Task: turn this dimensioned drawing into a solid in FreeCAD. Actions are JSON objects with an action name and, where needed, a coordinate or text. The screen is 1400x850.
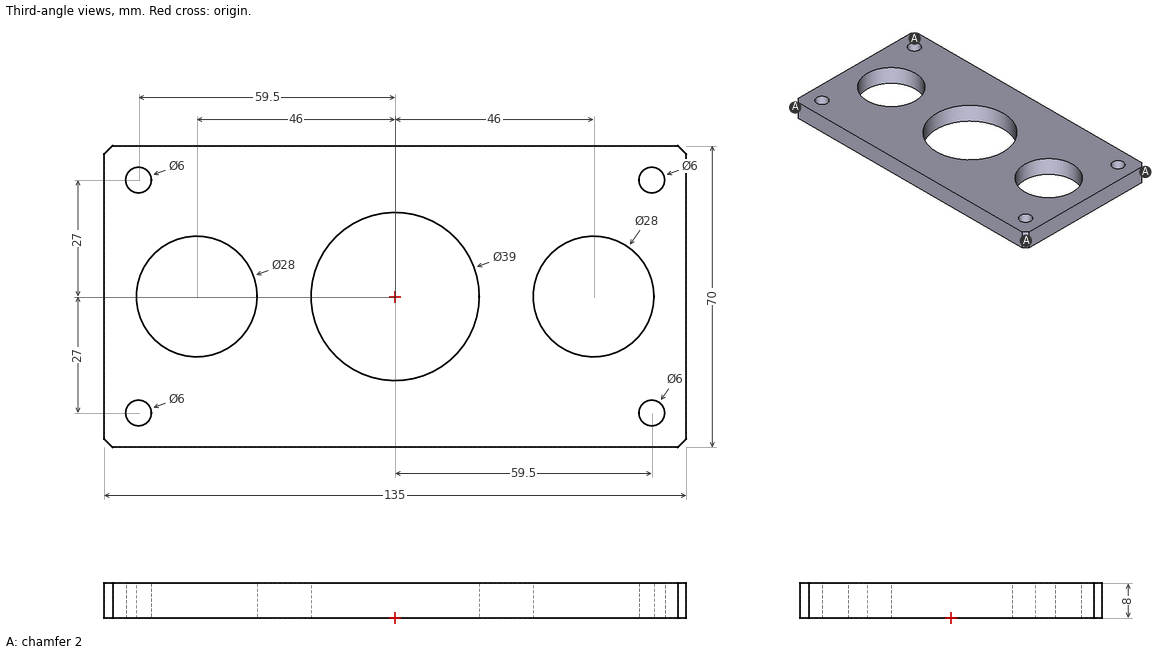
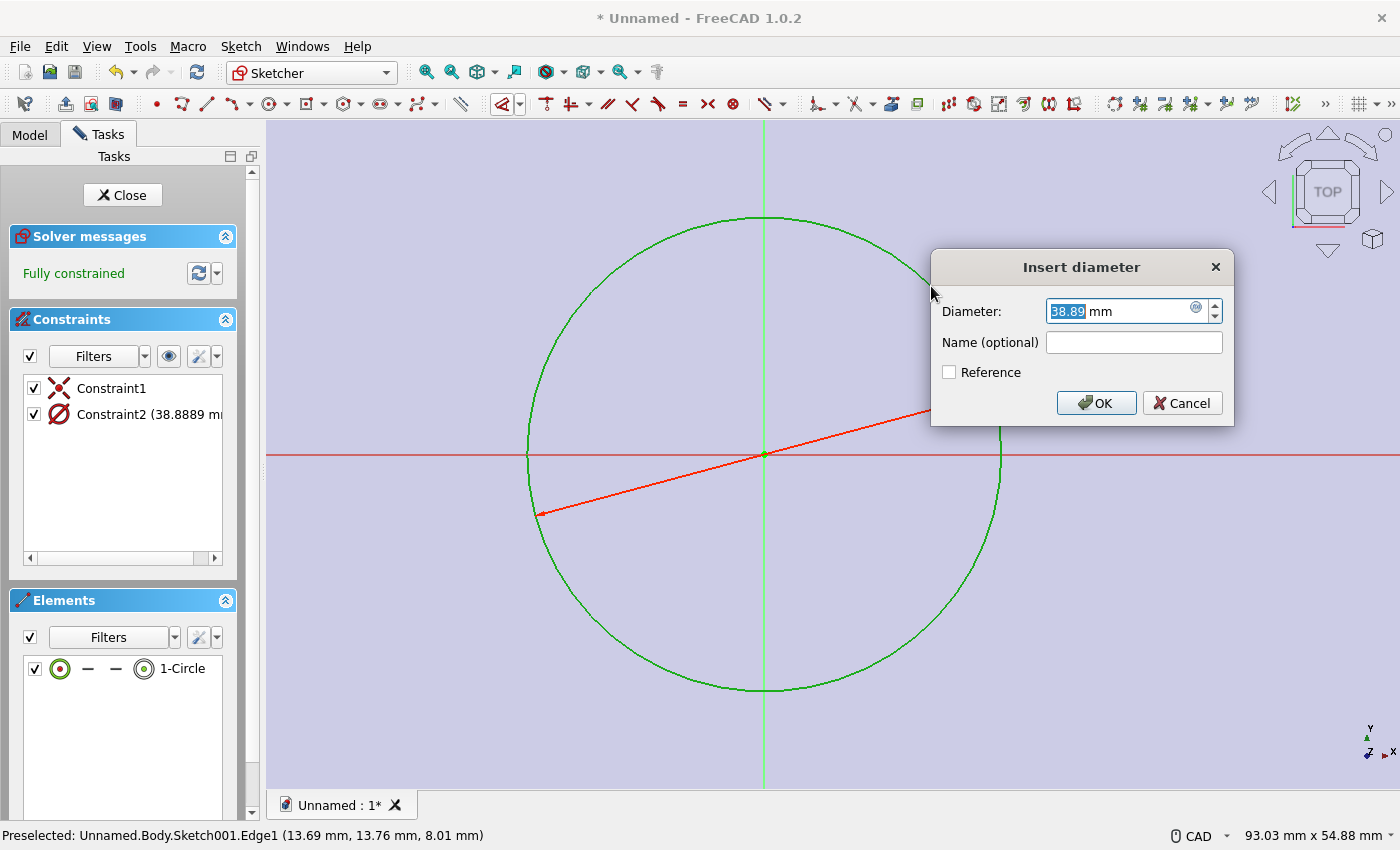
{"action": "type", "text": "39"}
{"action": "key", "text": "Return"}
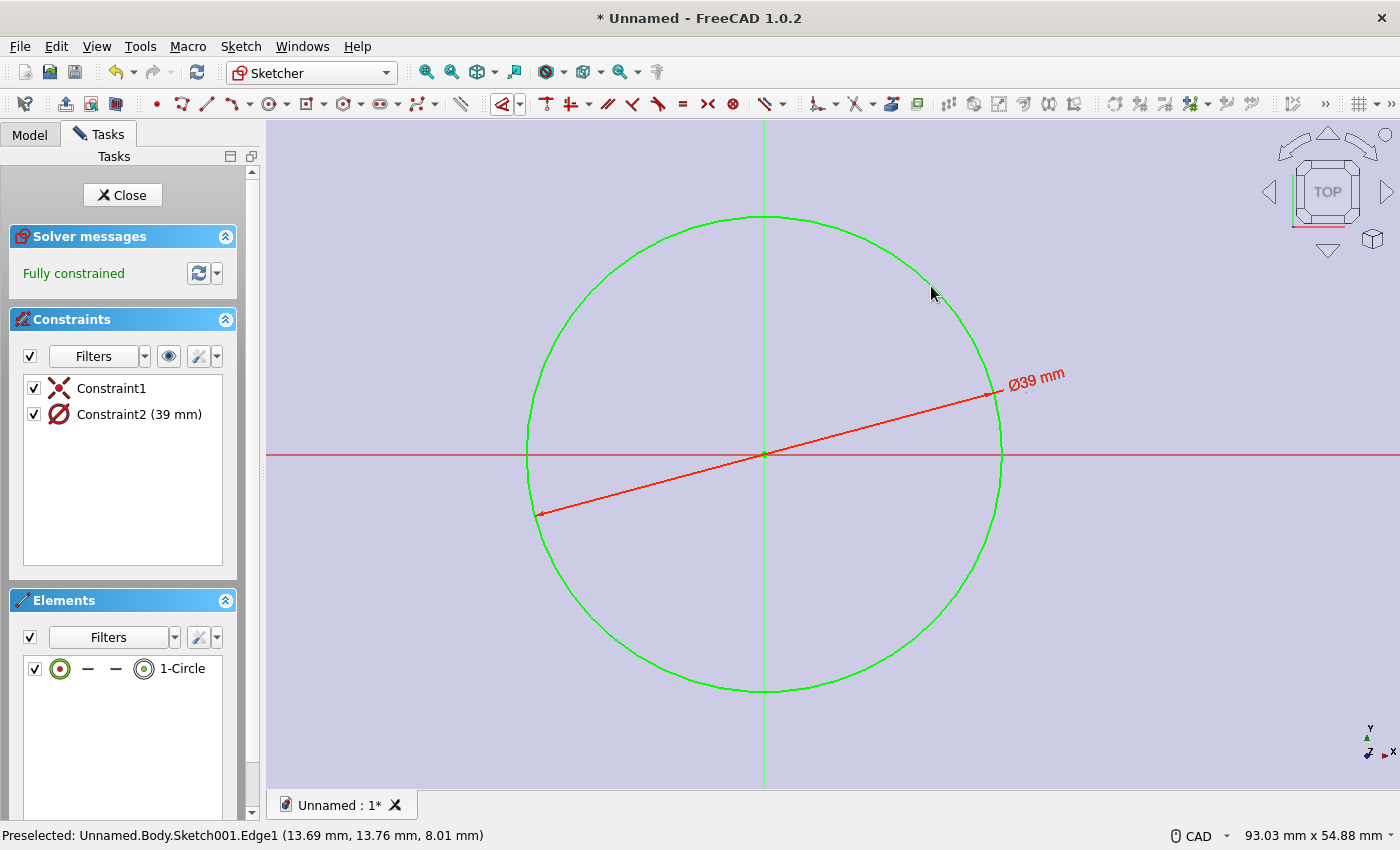
{"action": "left_click", "coordinate": [123, 195]}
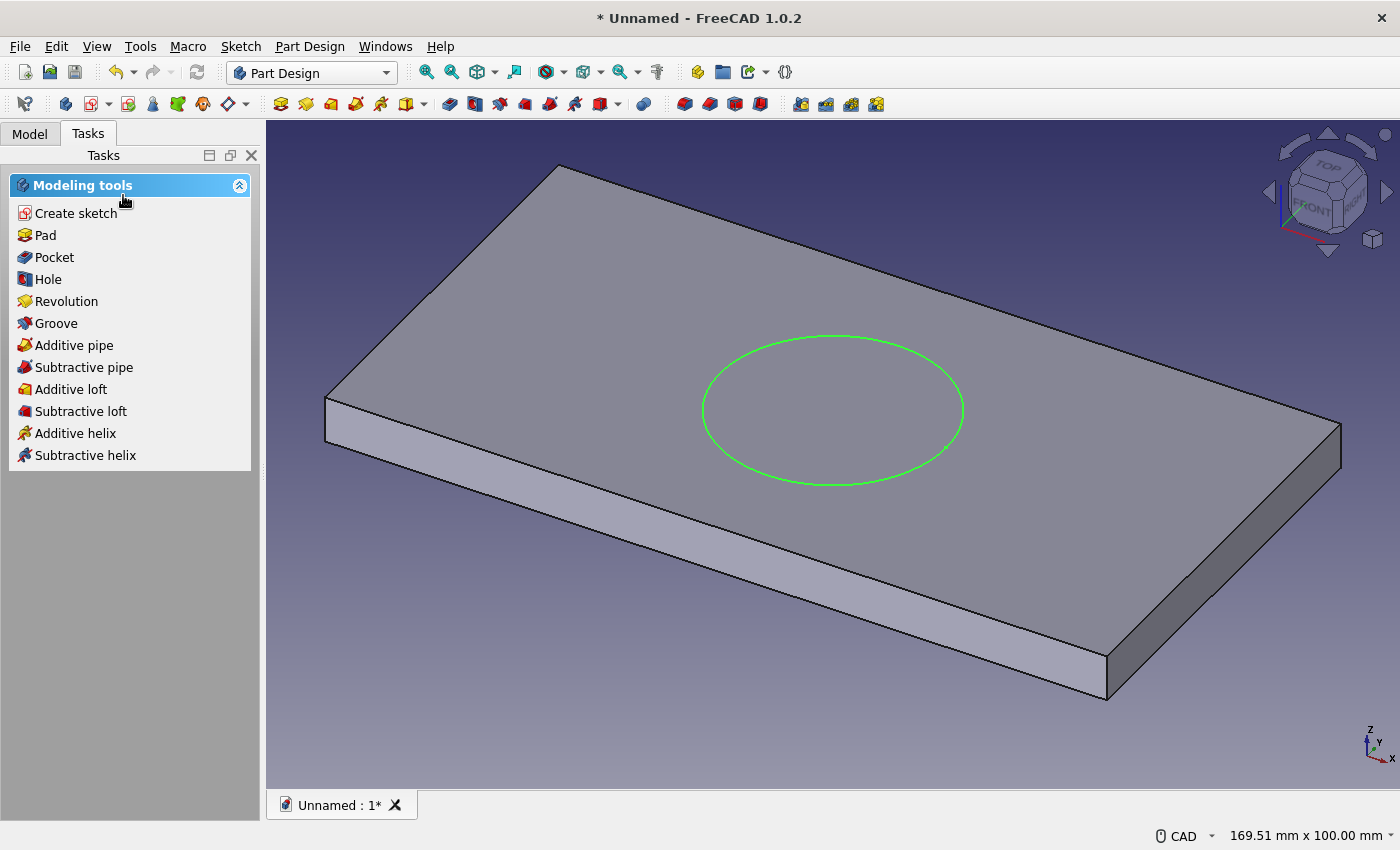
{"action": "left_click", "coordinate": [450, 104]}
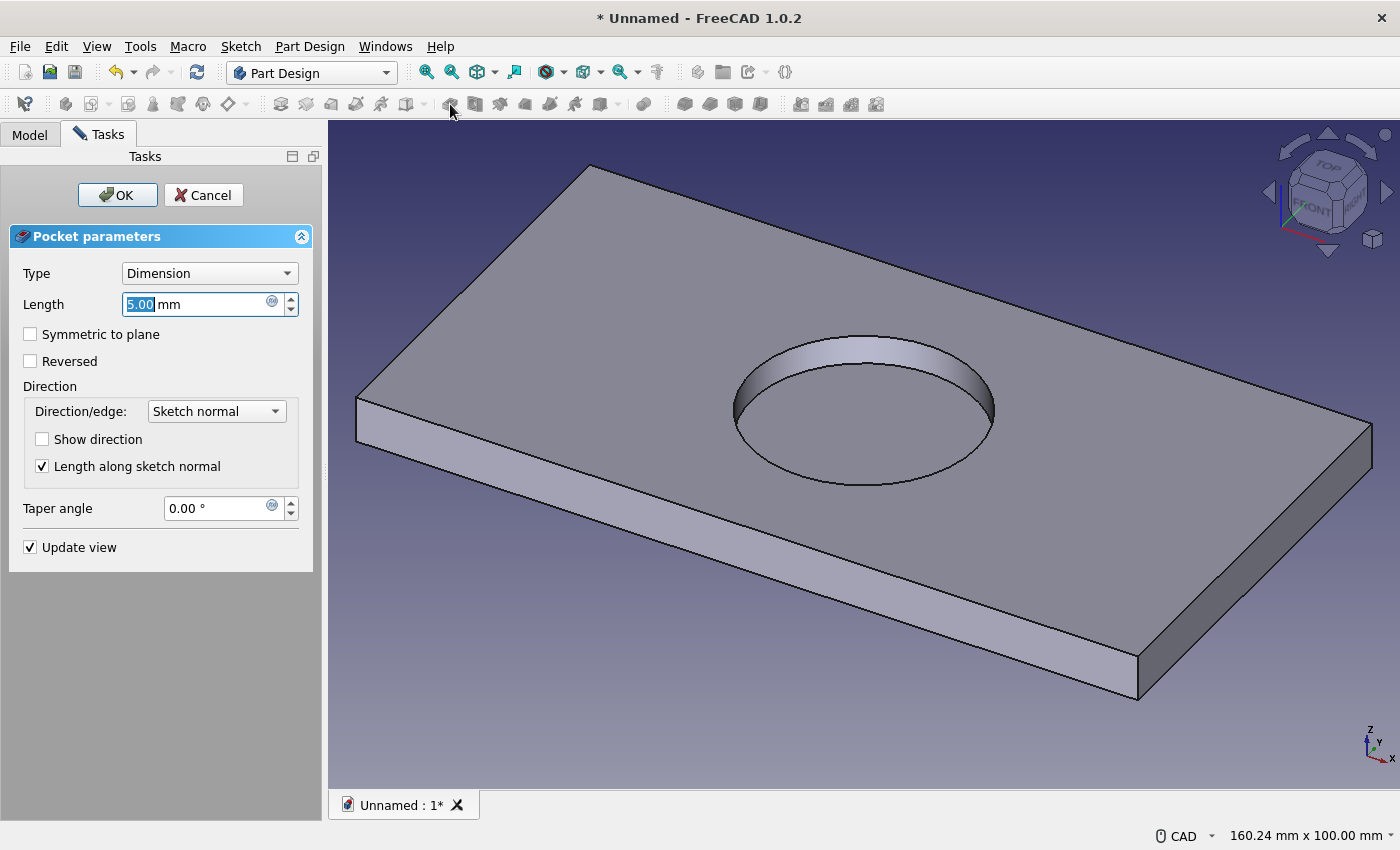
{"action": "left_click", "coordinate": [210, 274]}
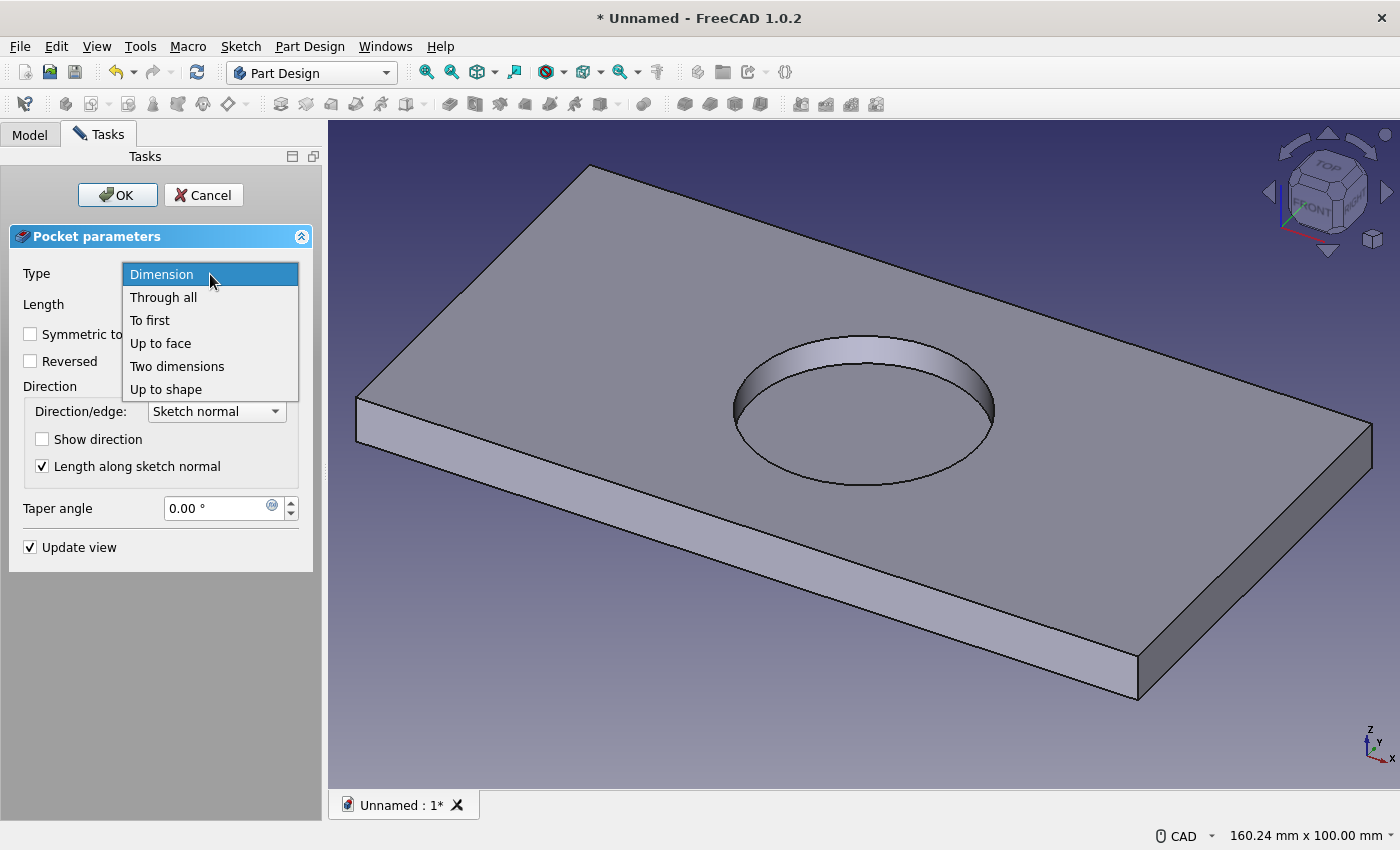
{"action": "left_click", "coordinate": [208, 320]}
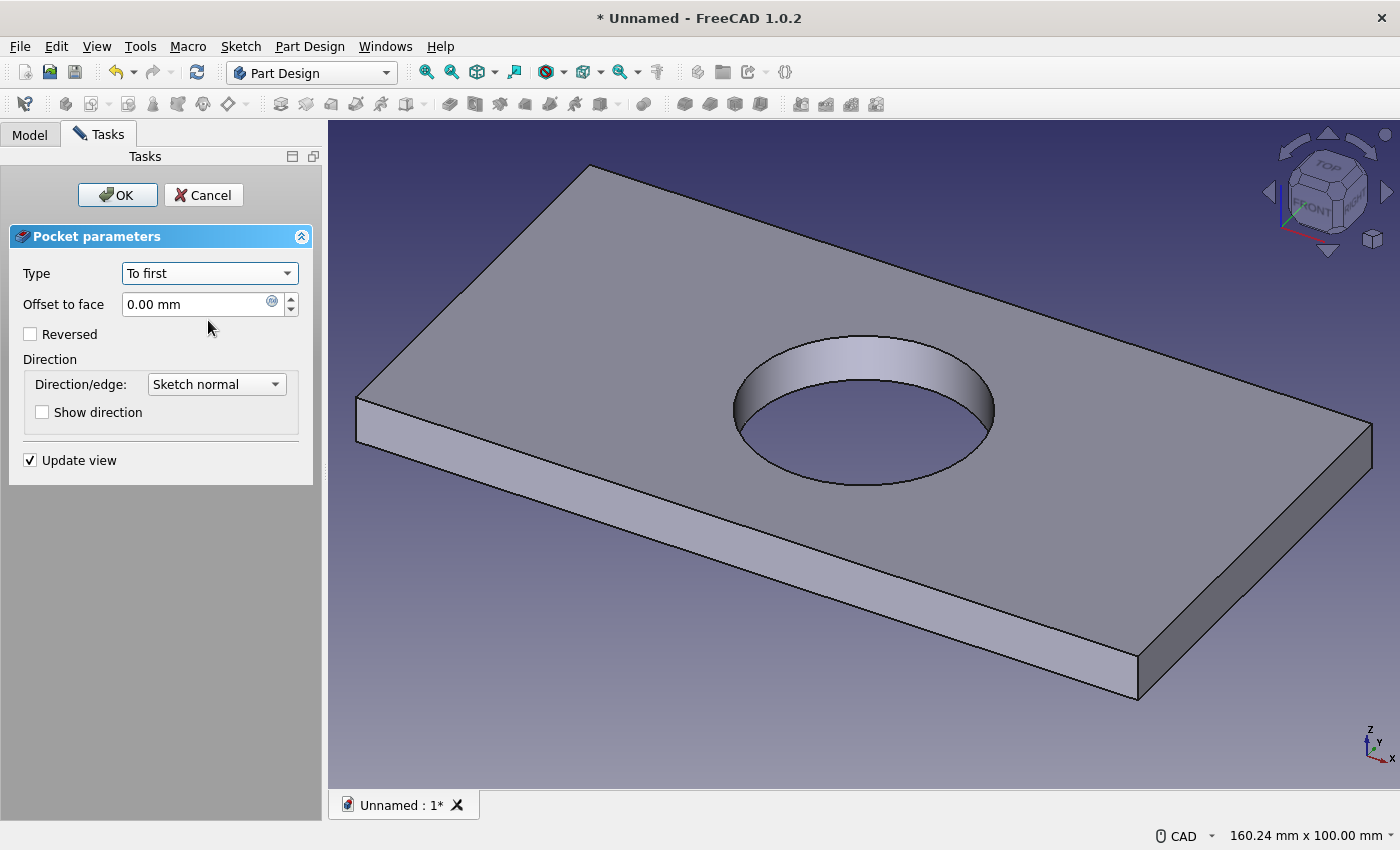
{"action": "left_click", "coordinate": [118, 195]}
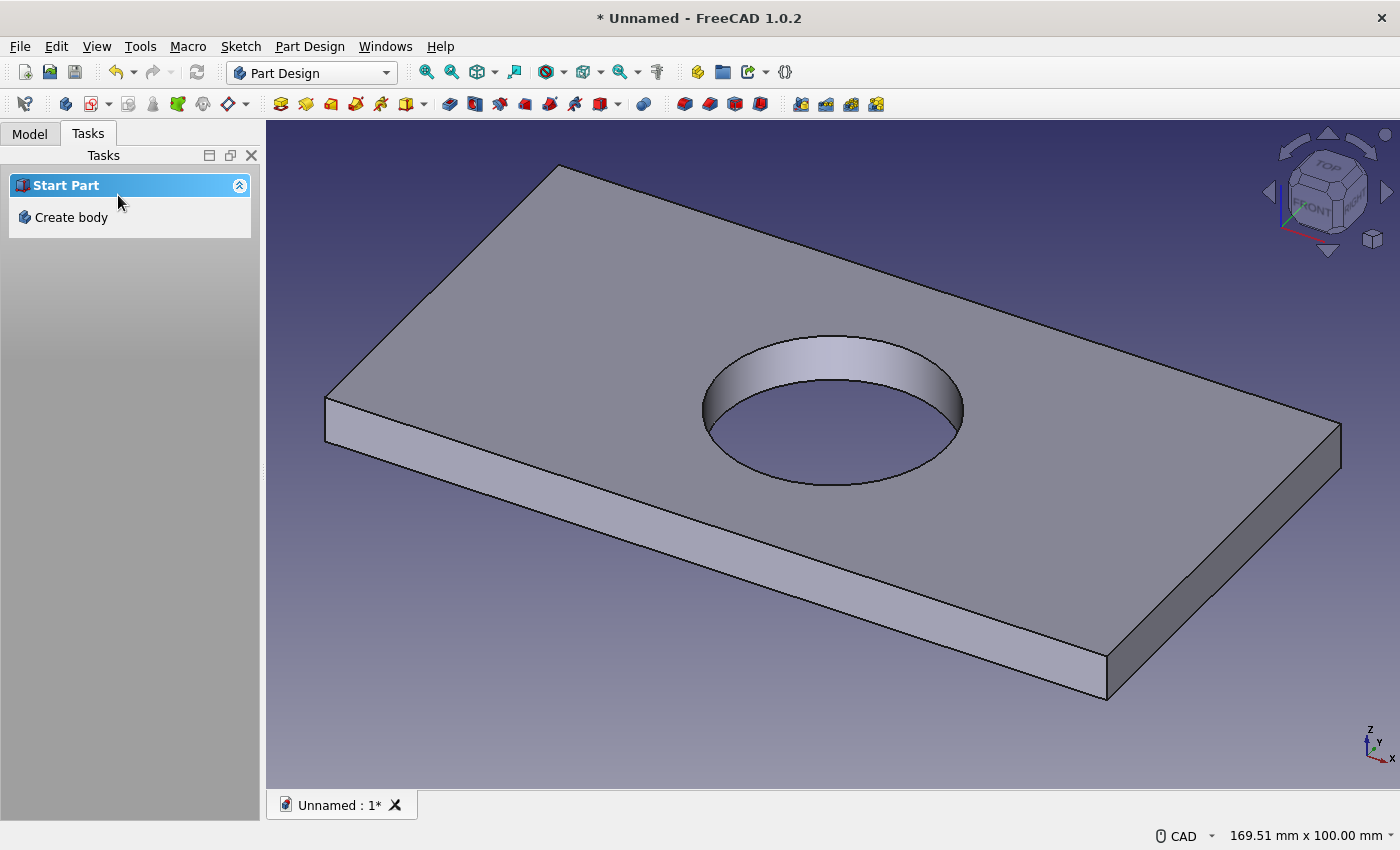
{"action": "left_click", "coordinate": [1023, 517]}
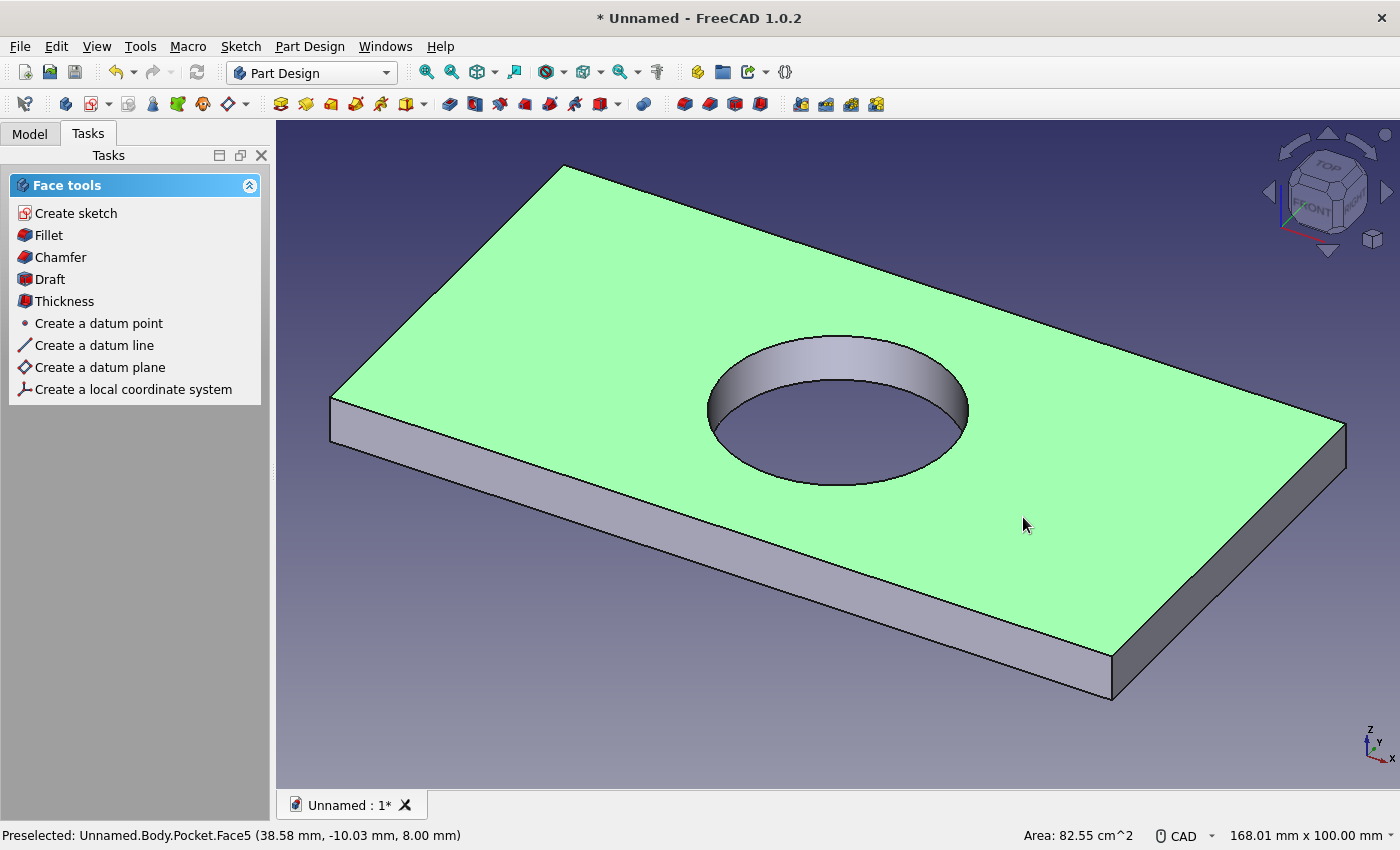
{"action": "left_click", "coordinate": [90, 104]}